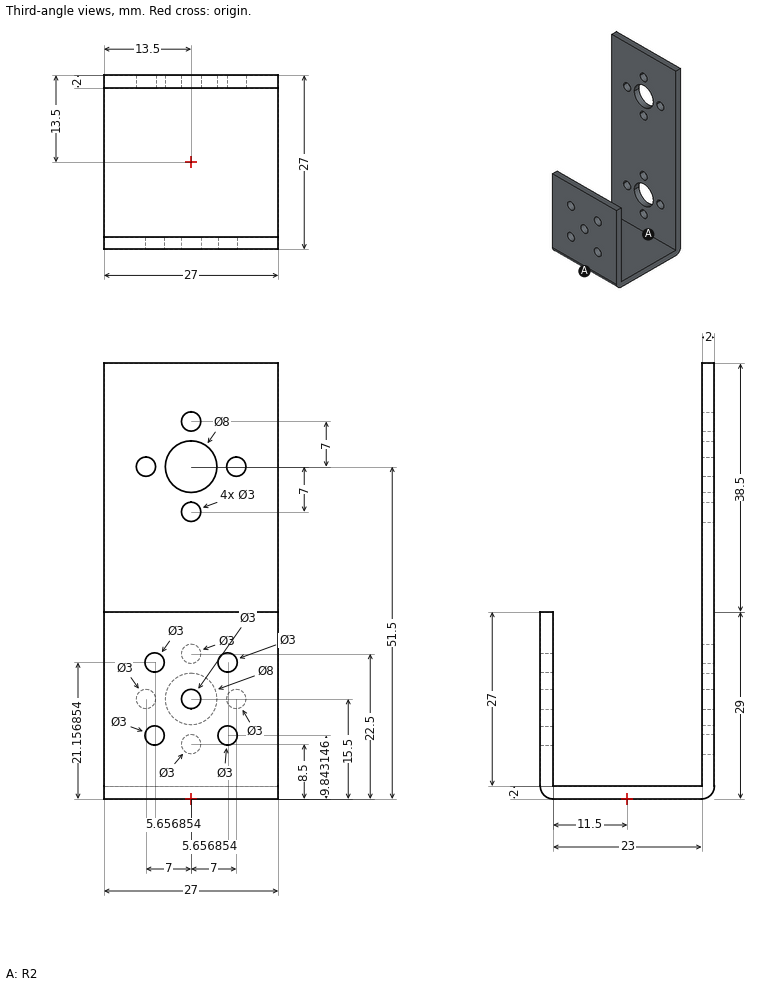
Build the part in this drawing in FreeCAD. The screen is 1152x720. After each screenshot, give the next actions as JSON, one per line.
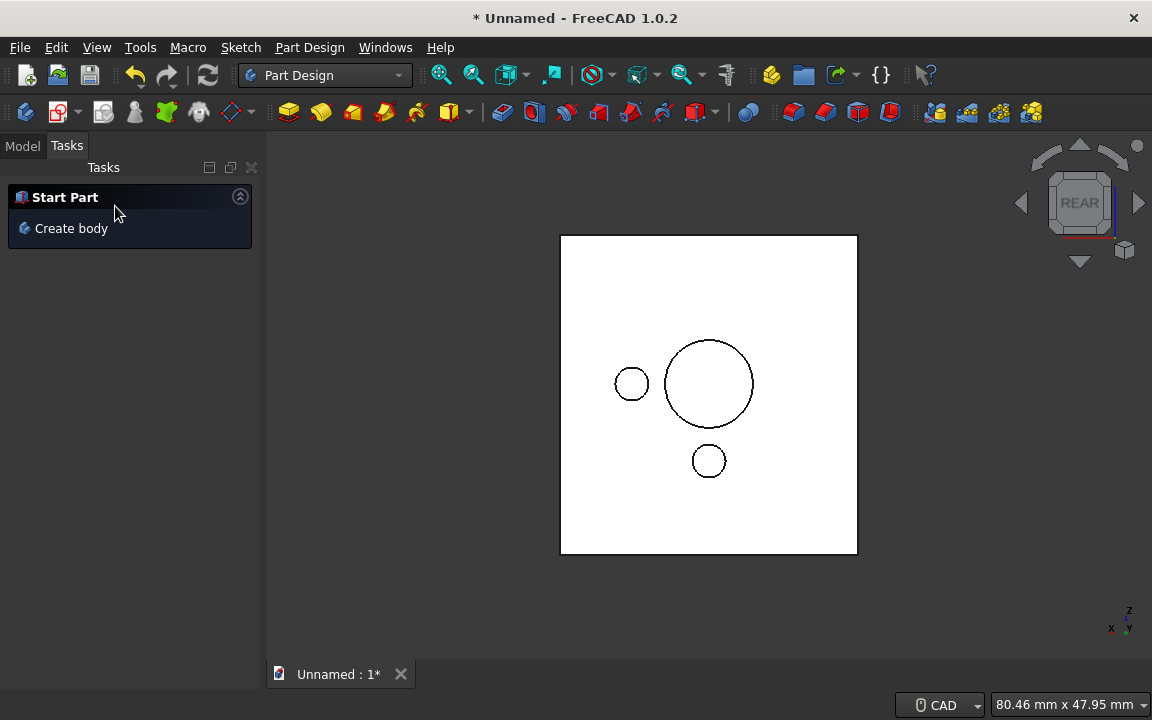
{"action": "left_click", "coordinate": [624, 303]}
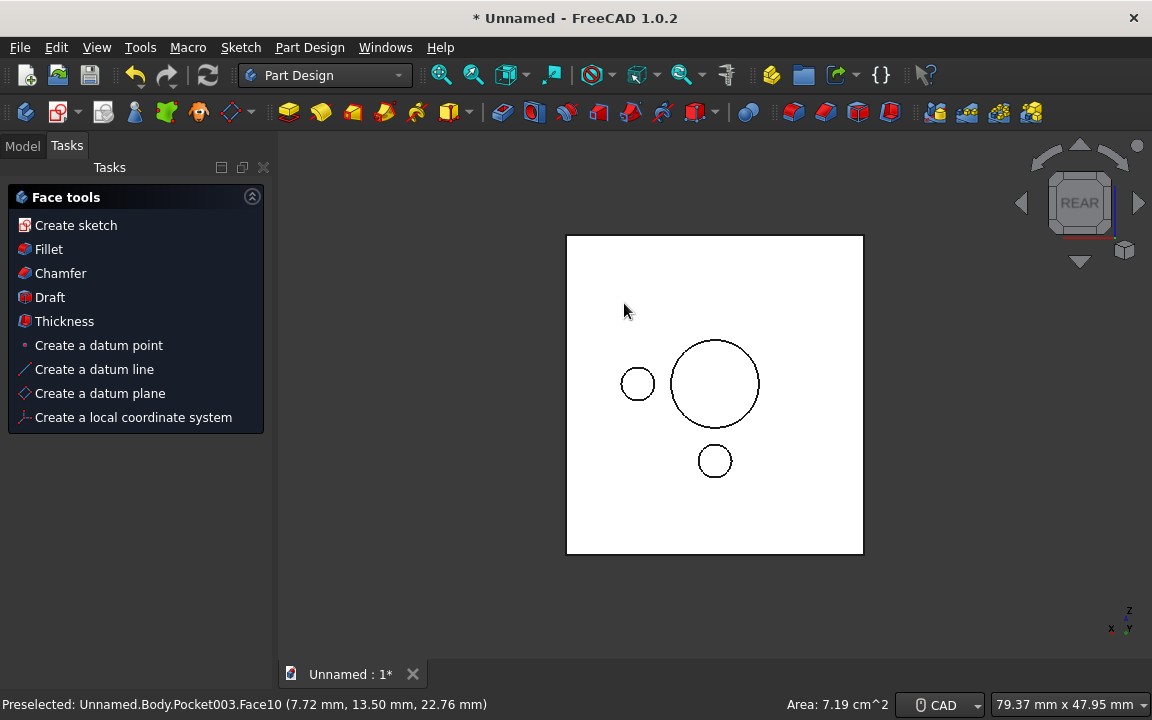
{"action": "left_click", "coordinate": [58, 112]}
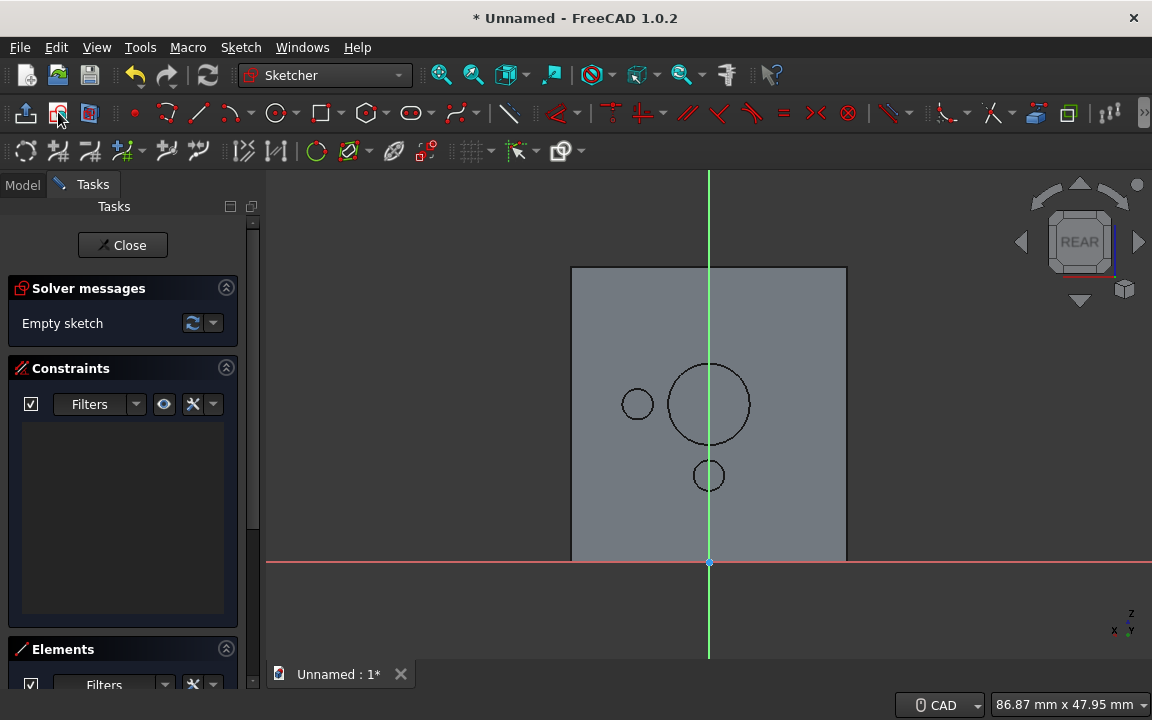
{"action": "scroll", "coordinate": [716, 325], "scroll_direction": "up", "scroll_amount": 12}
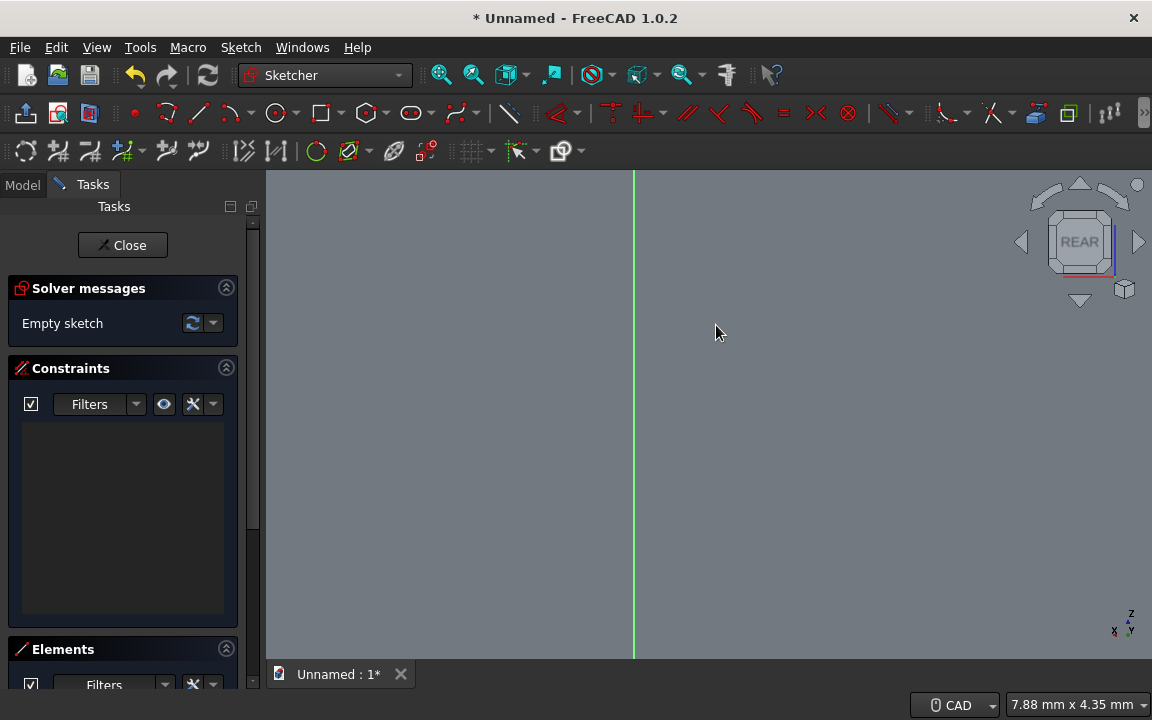
{"action": "key", "text": "g c"}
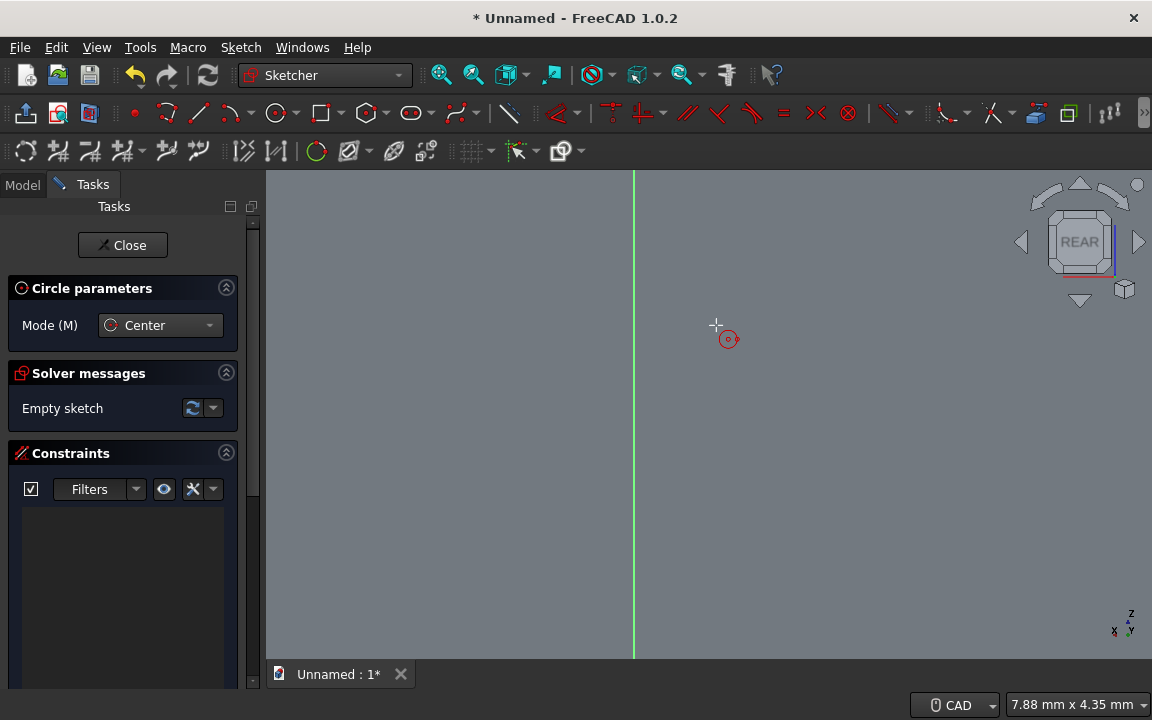
{"action": "left_click", "coordinate": [634, 409]}
{"action": "left_click", "coordinate": [753, 290]}
{"action": "key", "text": "Escape"}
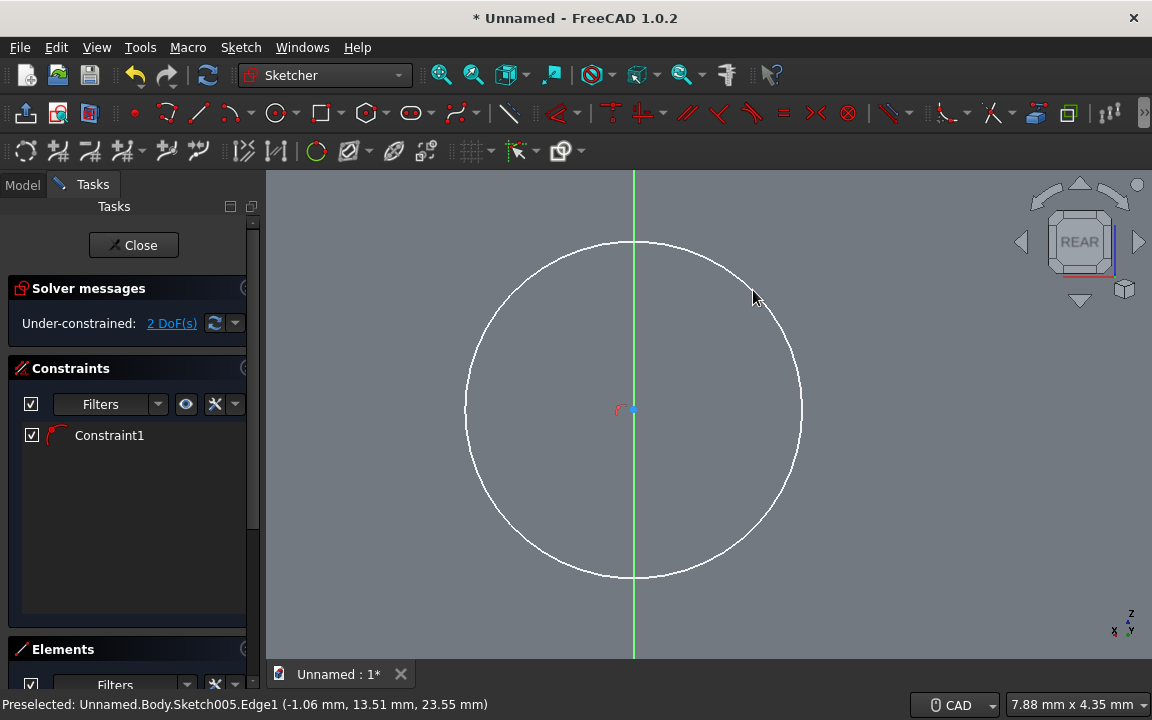
{"action": "key", "text": "d"}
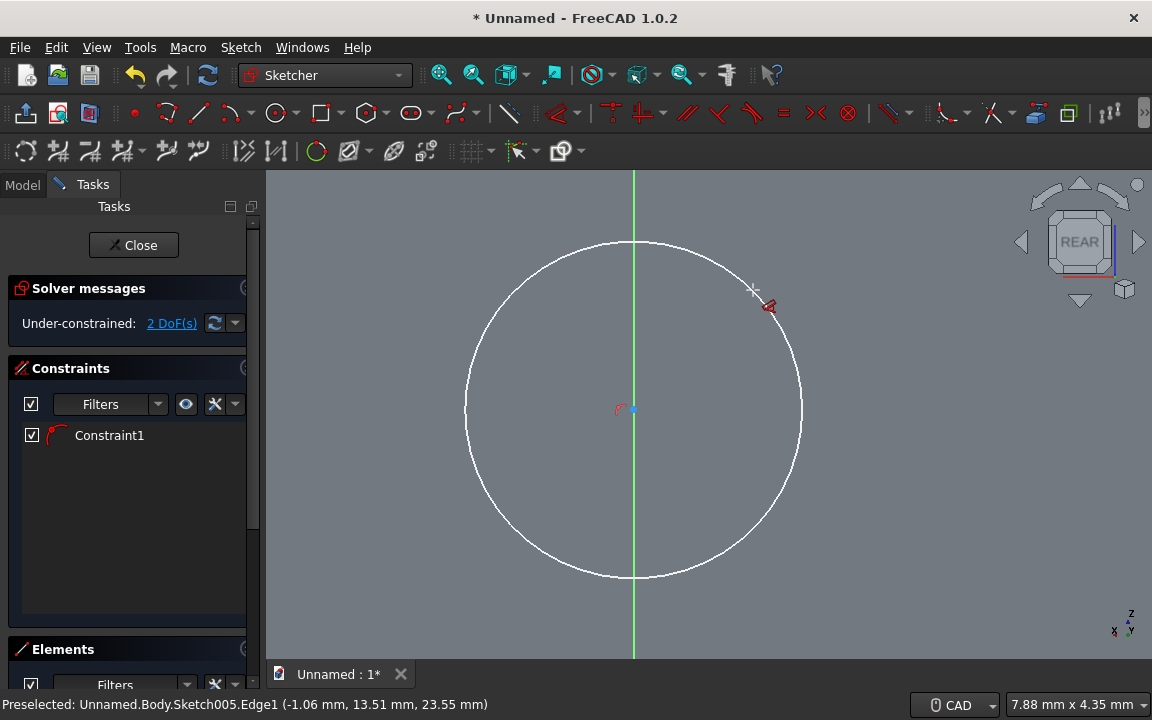
{"action": "left_click", "coordinate": [753, 291]}
{"action": "left_click", "coordinate": [776, 268]}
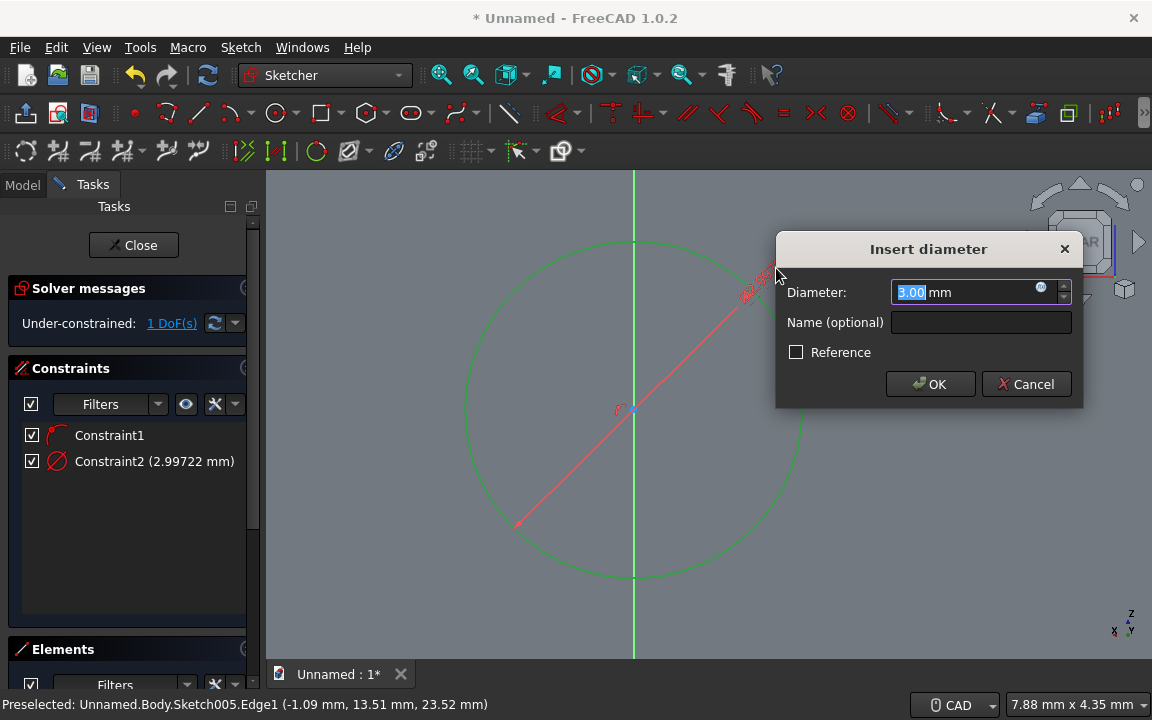
{"action": "type", "text": "3"}
{"action": "key", "text": "Return"}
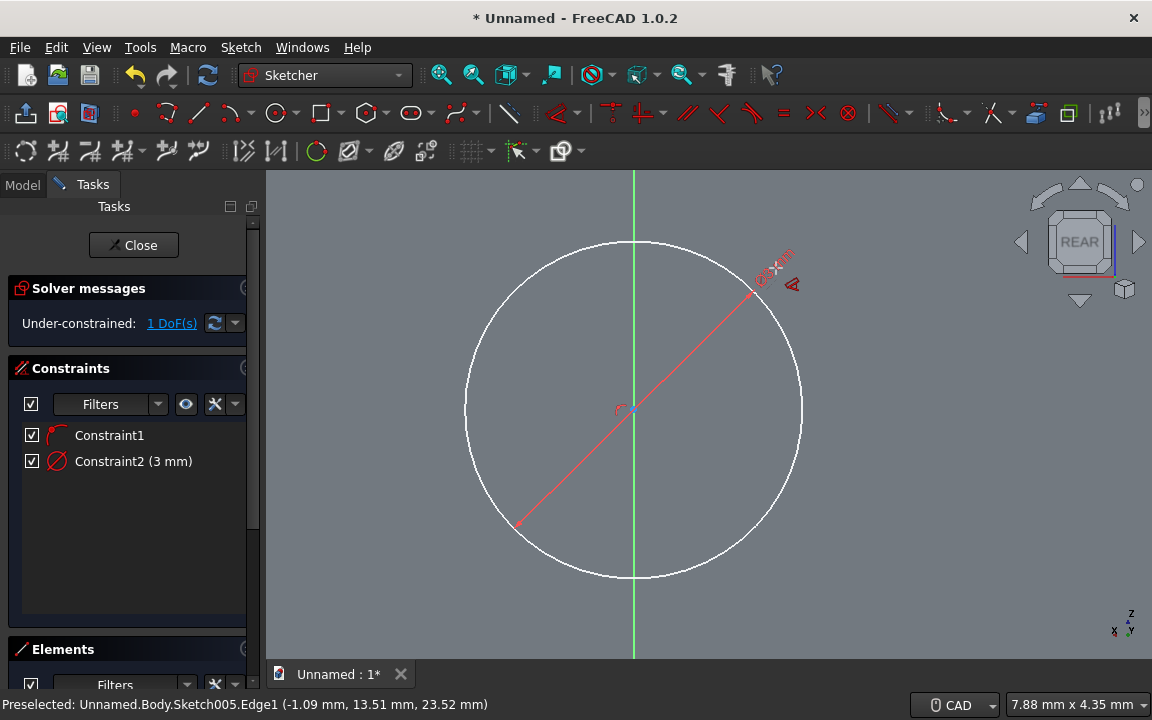
{"action": "left_click", "coordinate": [634, 410]}
{"action": "left_click", "coordinate": [668, 521]}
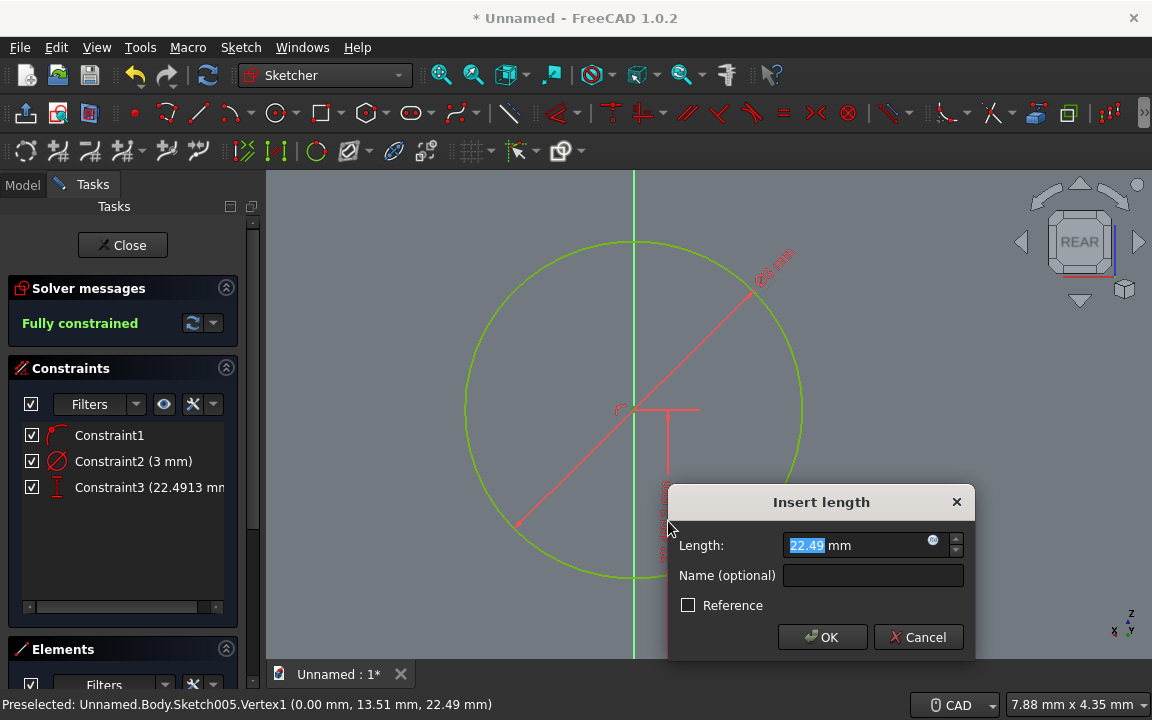
{"action": "type", "text": "22.5"}
{"action": "key", "text": "Return"}
{"action": "key", "text": "Escape"}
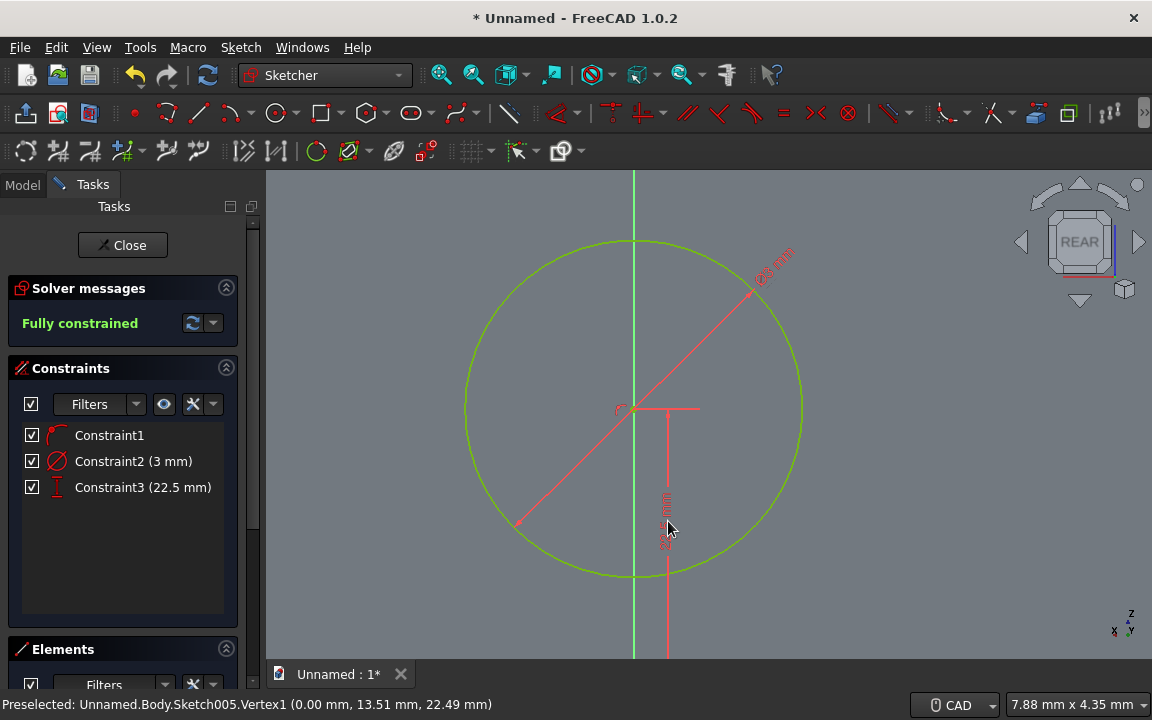
{"action": "left_click", "coordinate": [123, 245]}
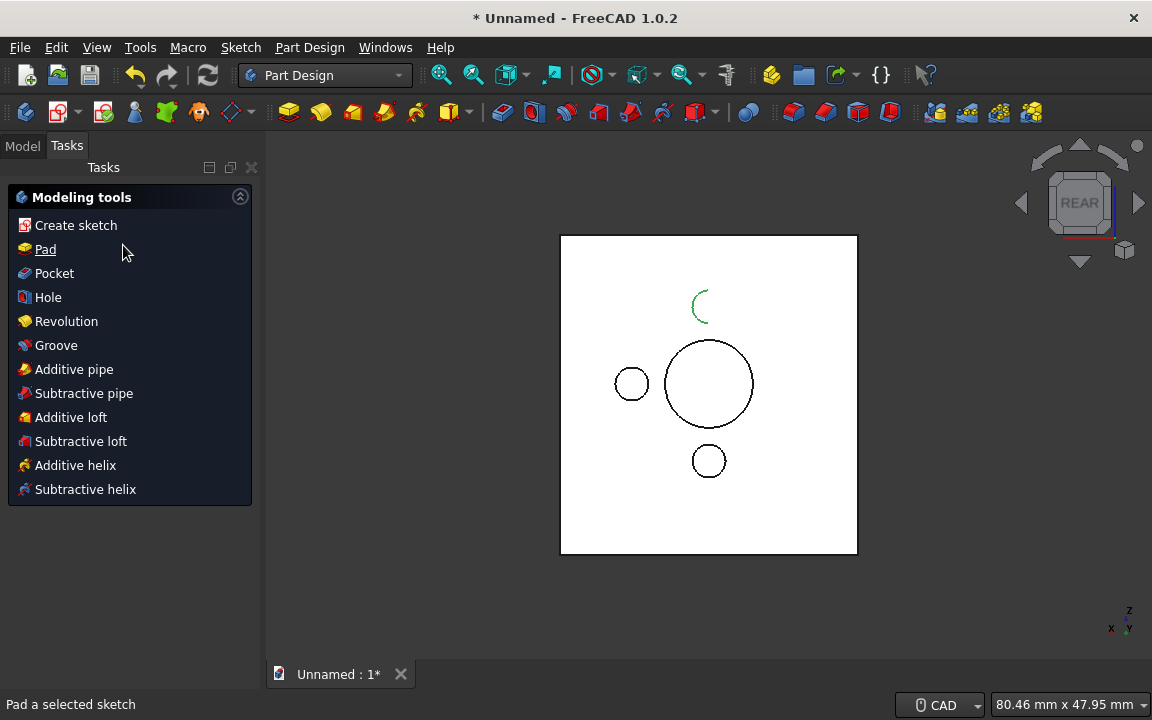
{"action": "left_click", "coordinate": [504, 112]}